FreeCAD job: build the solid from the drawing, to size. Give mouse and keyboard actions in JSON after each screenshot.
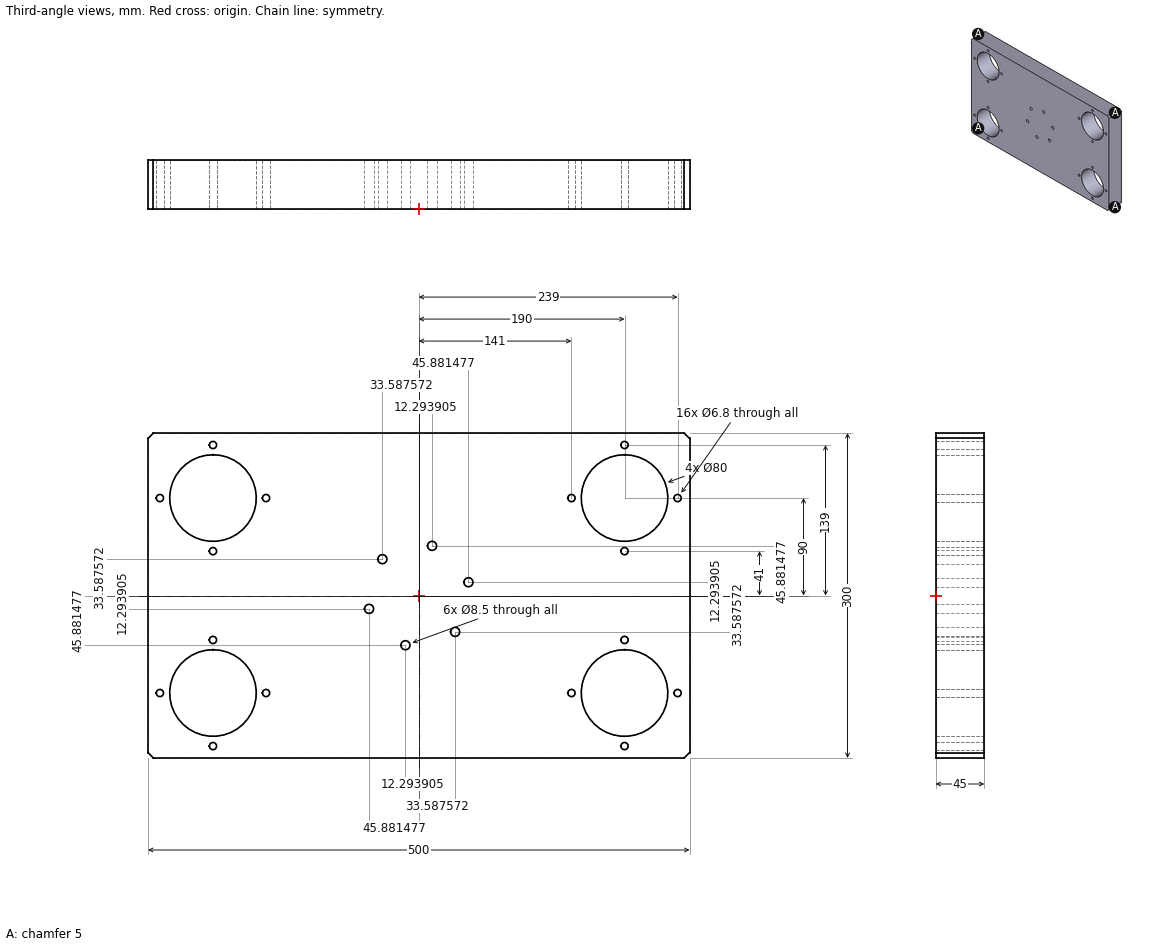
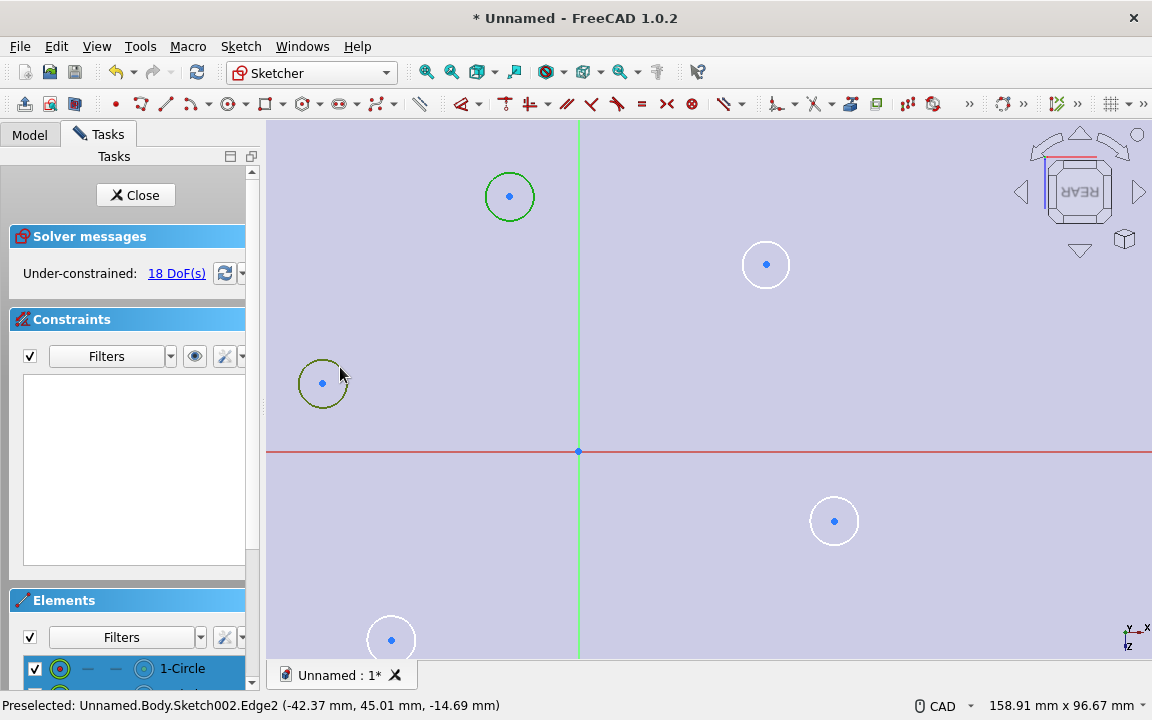
{"action": "left_click", "coordinate": [408, 623]}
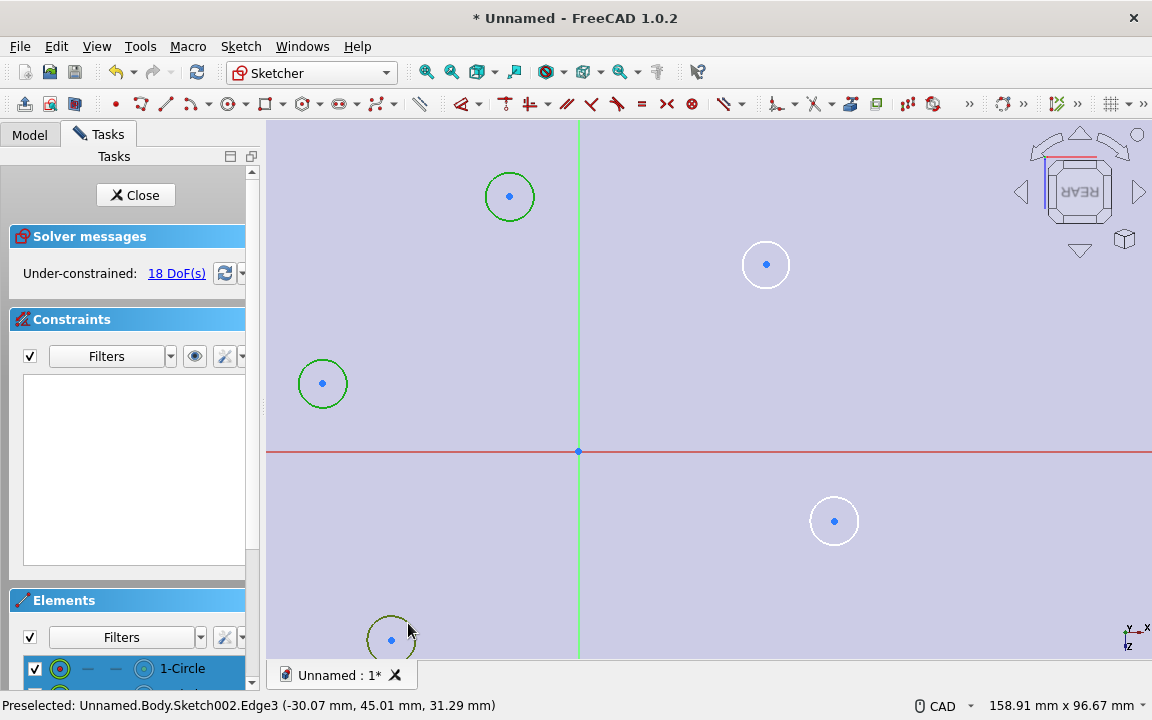
{"action": "scroll", "coordinate": [767, 263], "scroll_direction": "down", "scroll_amount": 2}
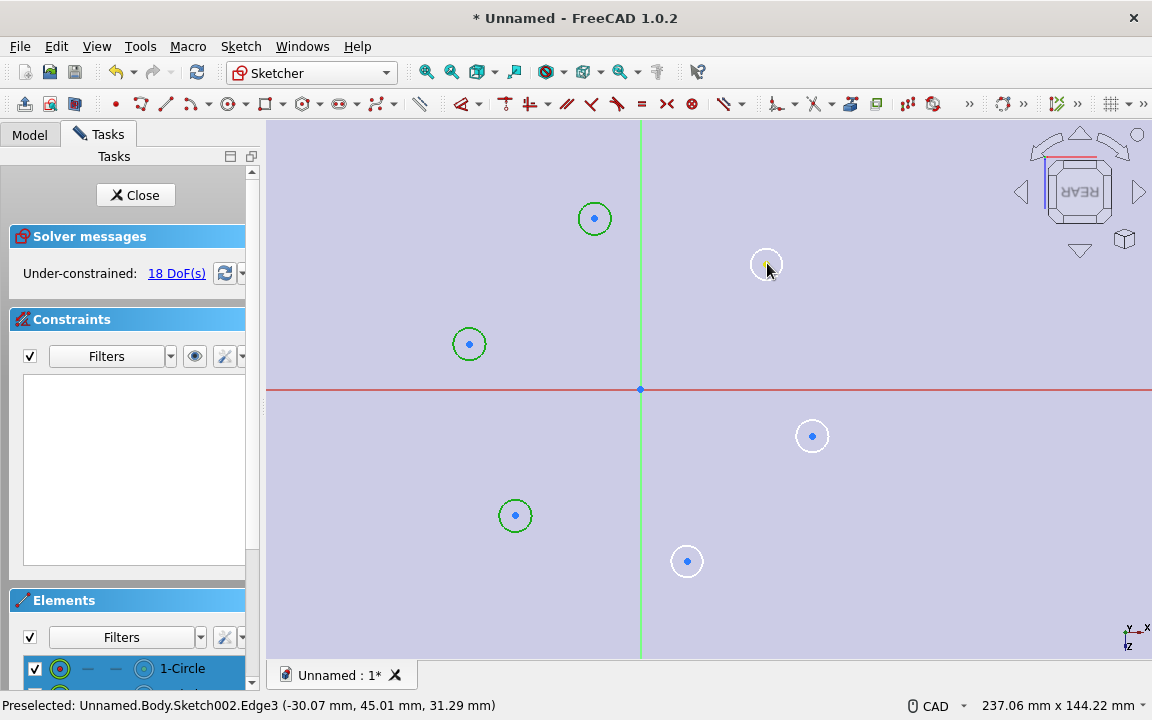
{"action": "left_click", "coordinate": [698, 550]}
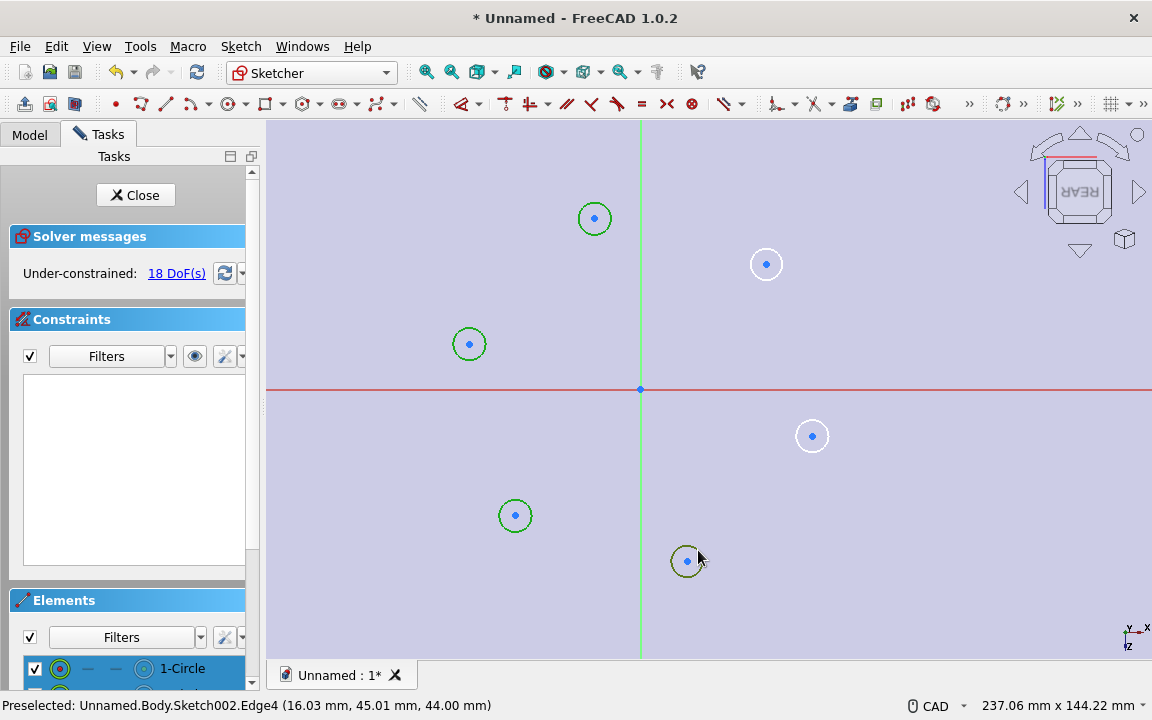
{"action": "left_click", "coordinate": [824, 425]}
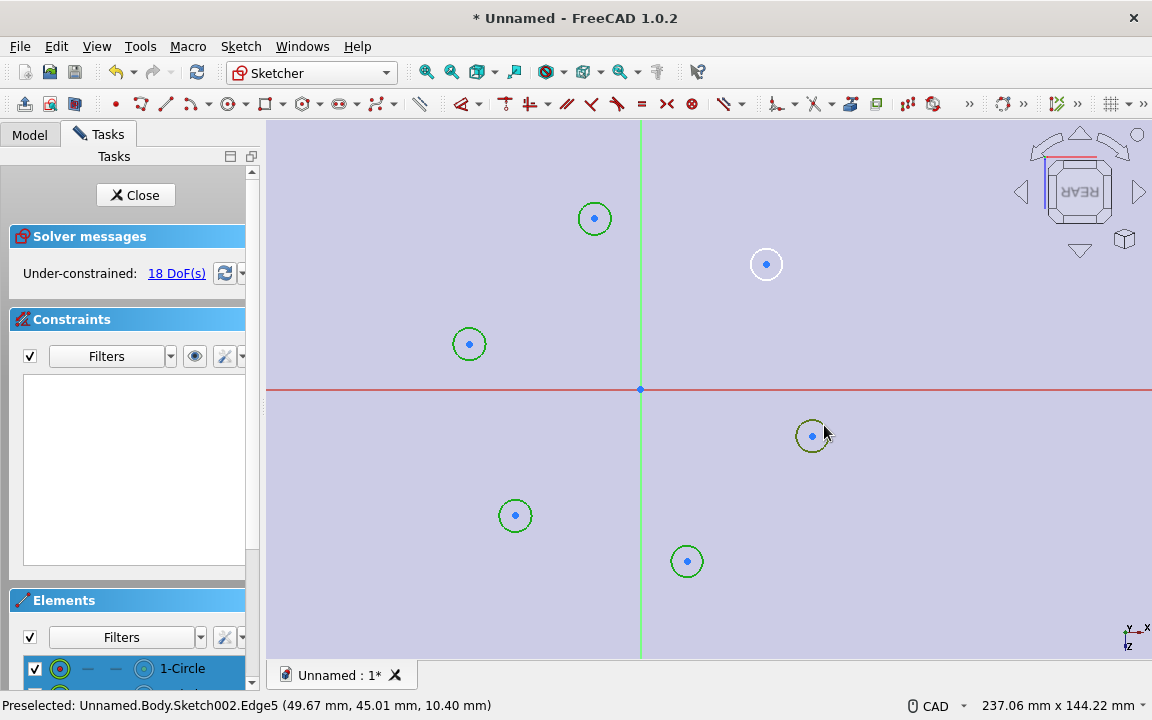
{"action": "left_click", "coordinate": [778, 253]}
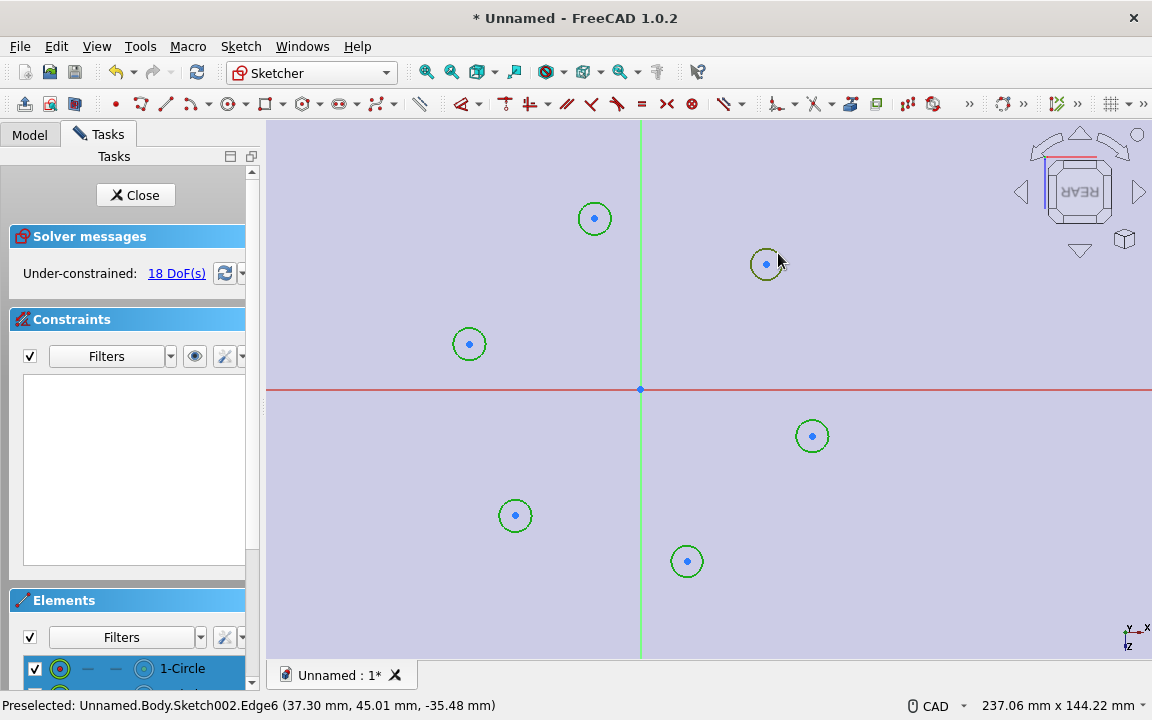
{"action": "left_click", "coordinate": [642, 104]}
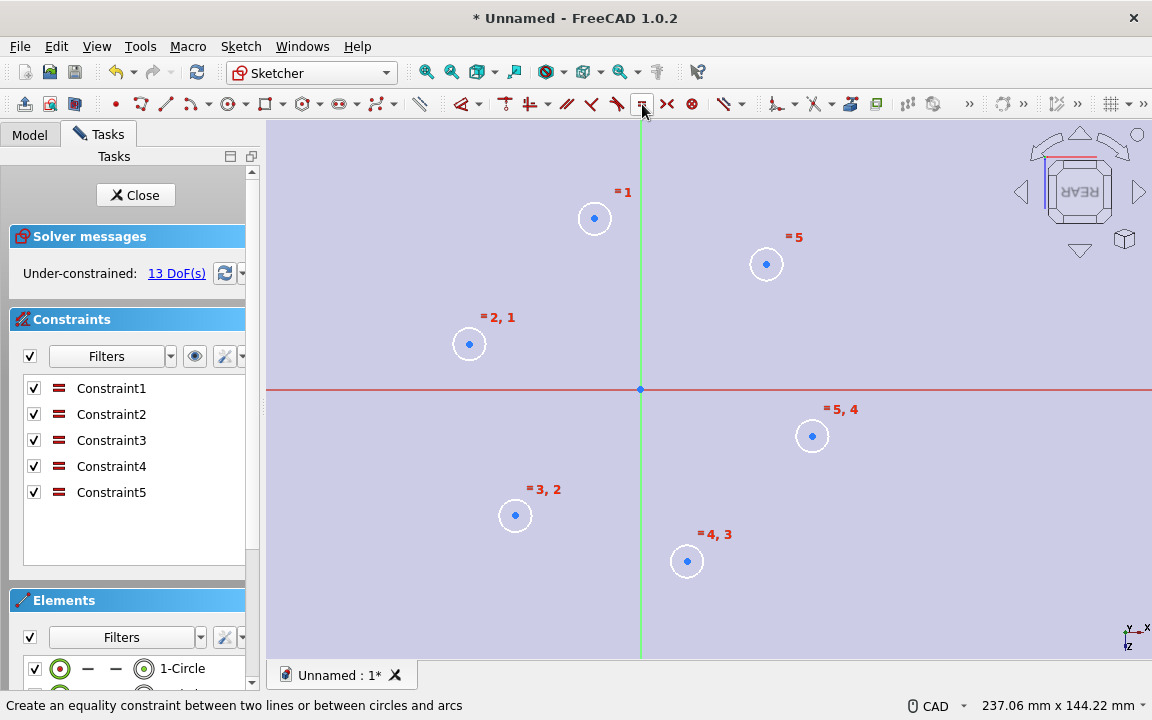
{"action": "left_click", "coordinate": [460, 104]}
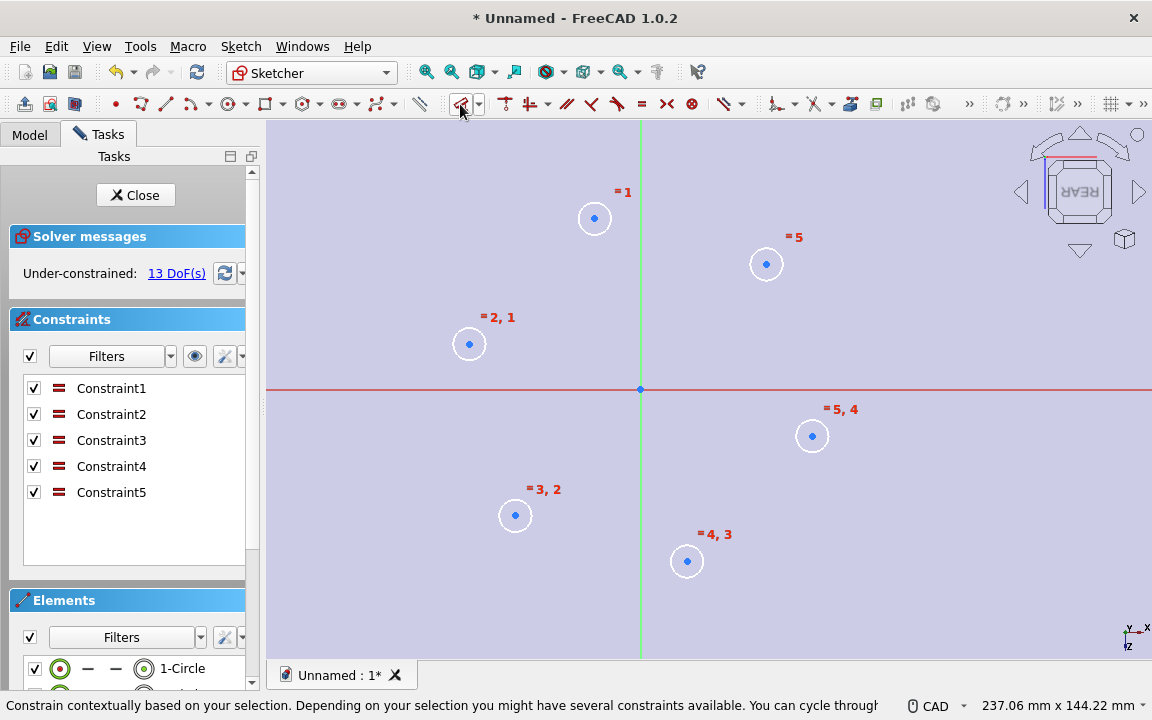
{"action": "scroll", "coordinate": [606, 207], "scroll_direction": "up", "scroll_amount": 2}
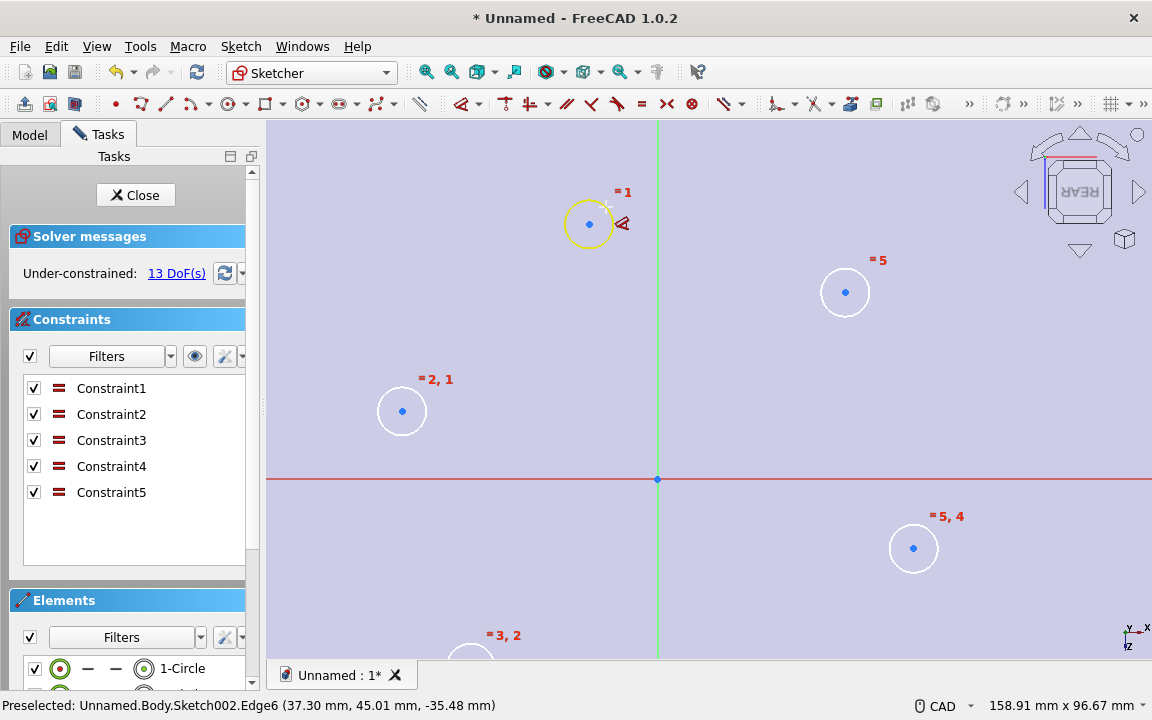
{"action": "left_click", "coordinate": [606, 207]}
{"action": "left_click", "coordinate": [628, 184]}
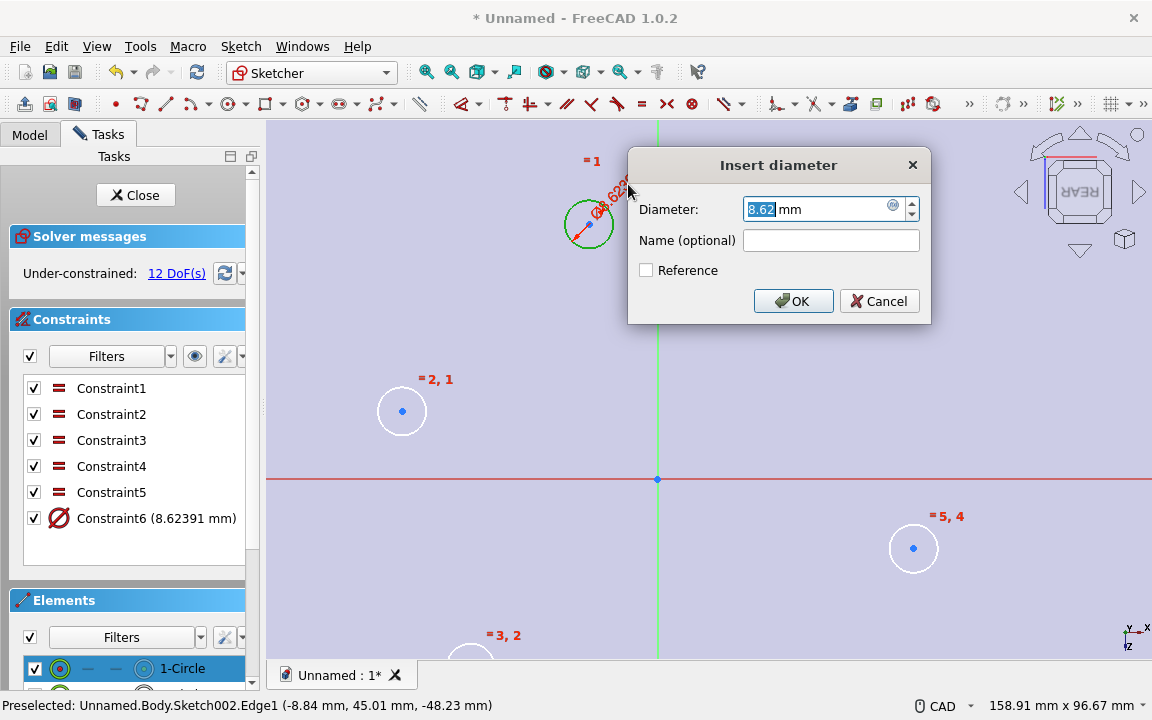
{"action": "type", "text": "8.5"}
{"action": "key", "text": "Return"}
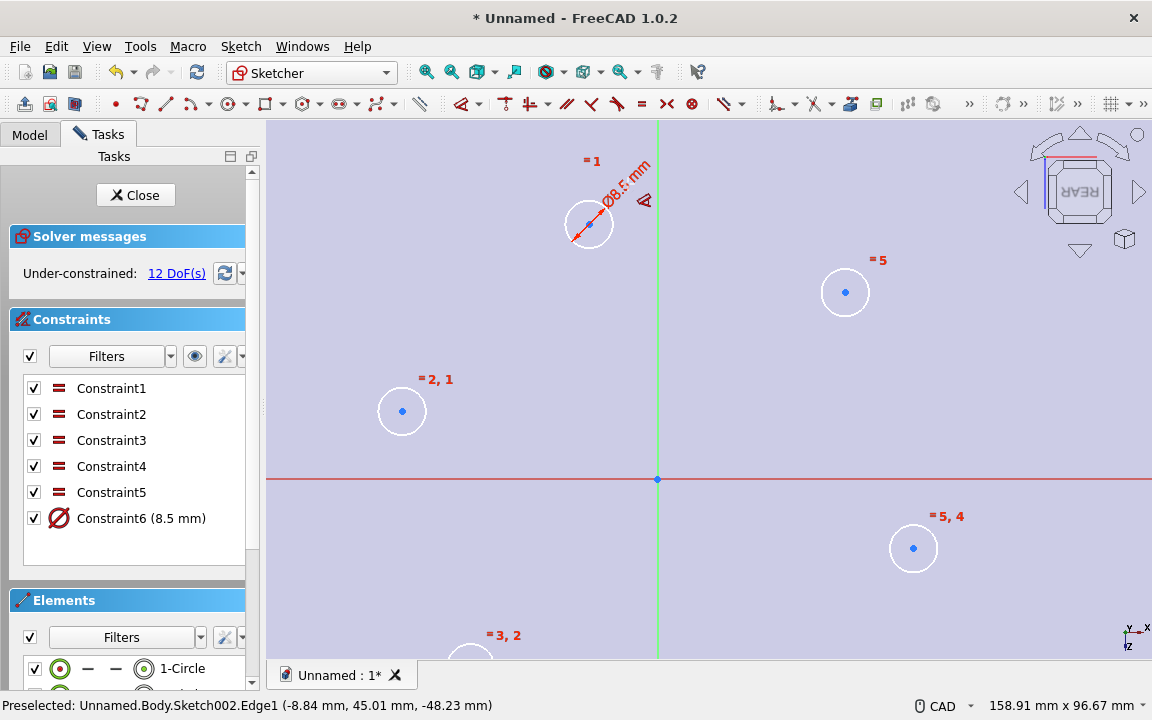
{"action": "left_click", "coordinate": [589, 224]}
{"action": "left_click", "coordinate": [623, 513]}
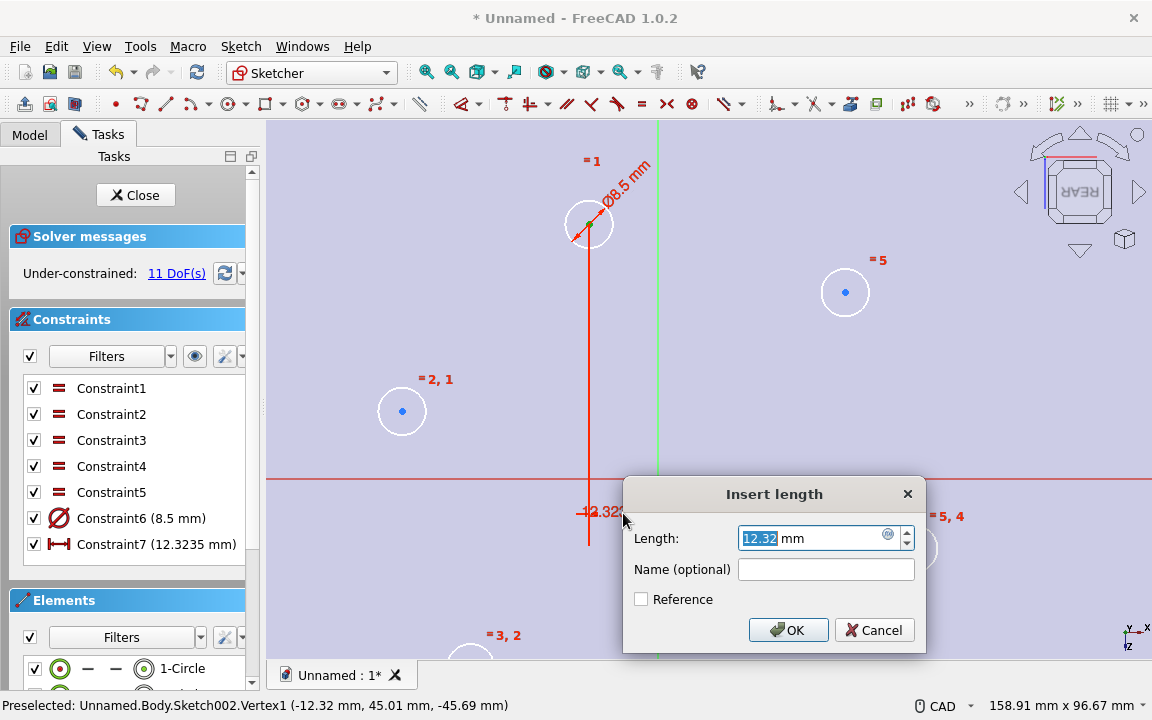
{"action": "type", "text": "12.293905"}
{"action": "key", "text": "Return"}